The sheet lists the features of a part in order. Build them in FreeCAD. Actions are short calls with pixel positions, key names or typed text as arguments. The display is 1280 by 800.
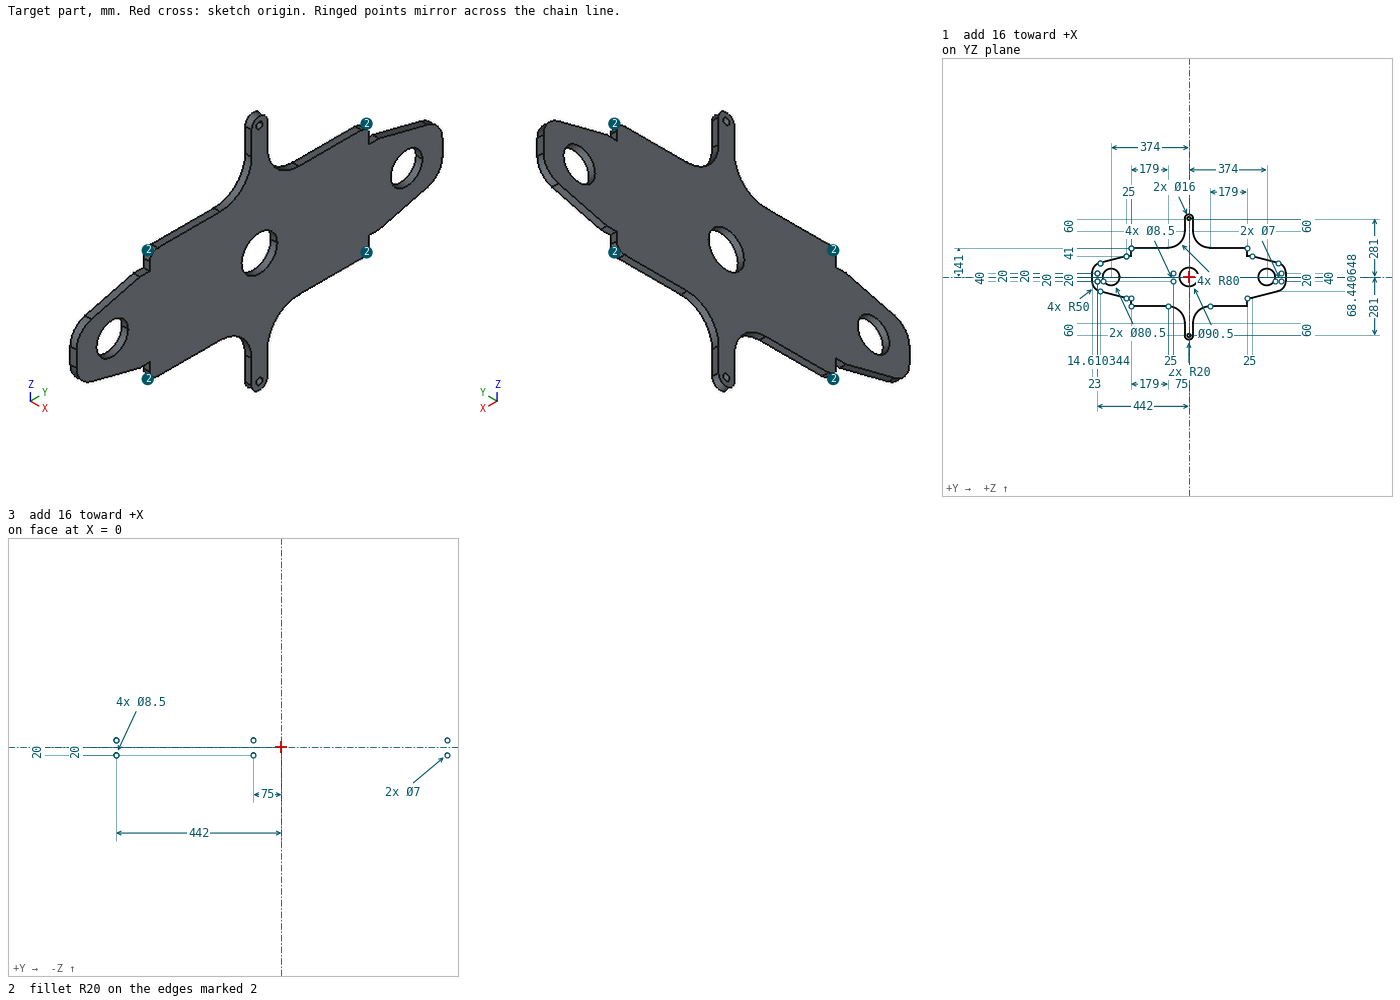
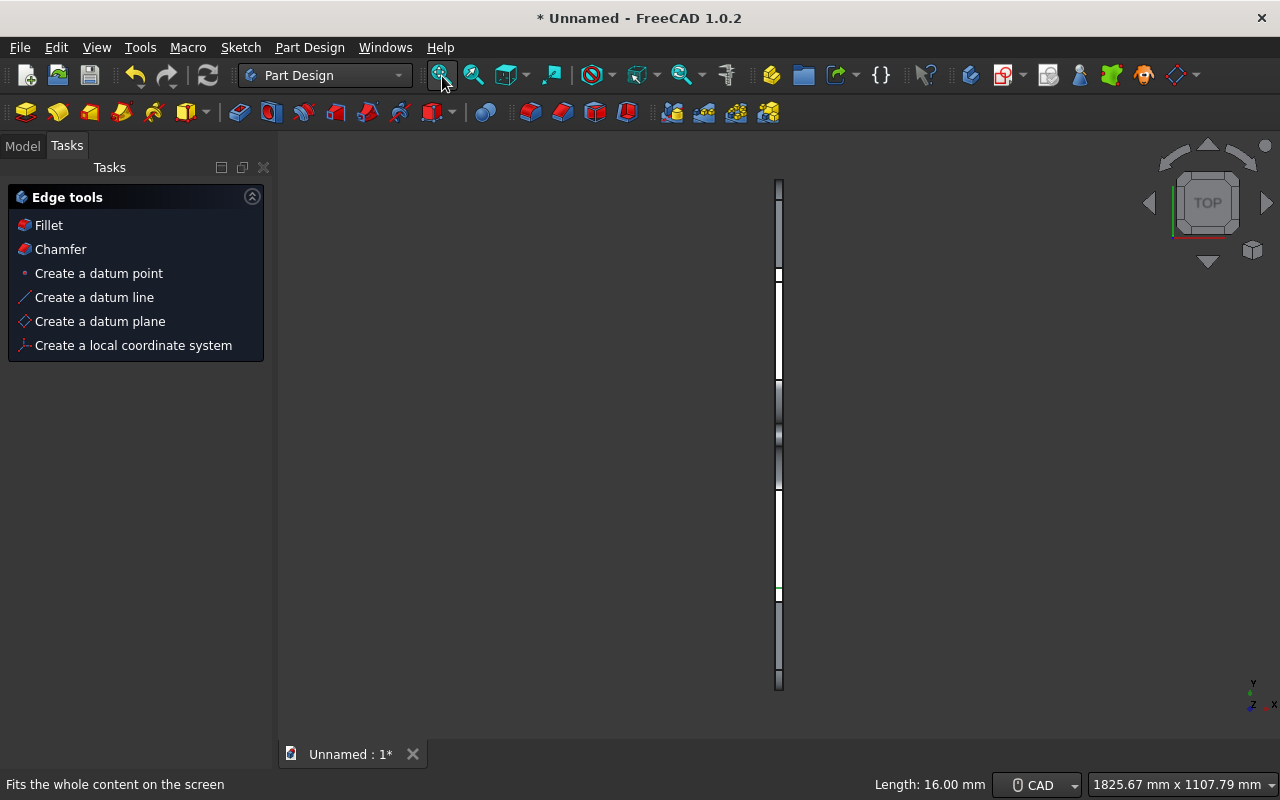
scroll(779, 281, up, 8)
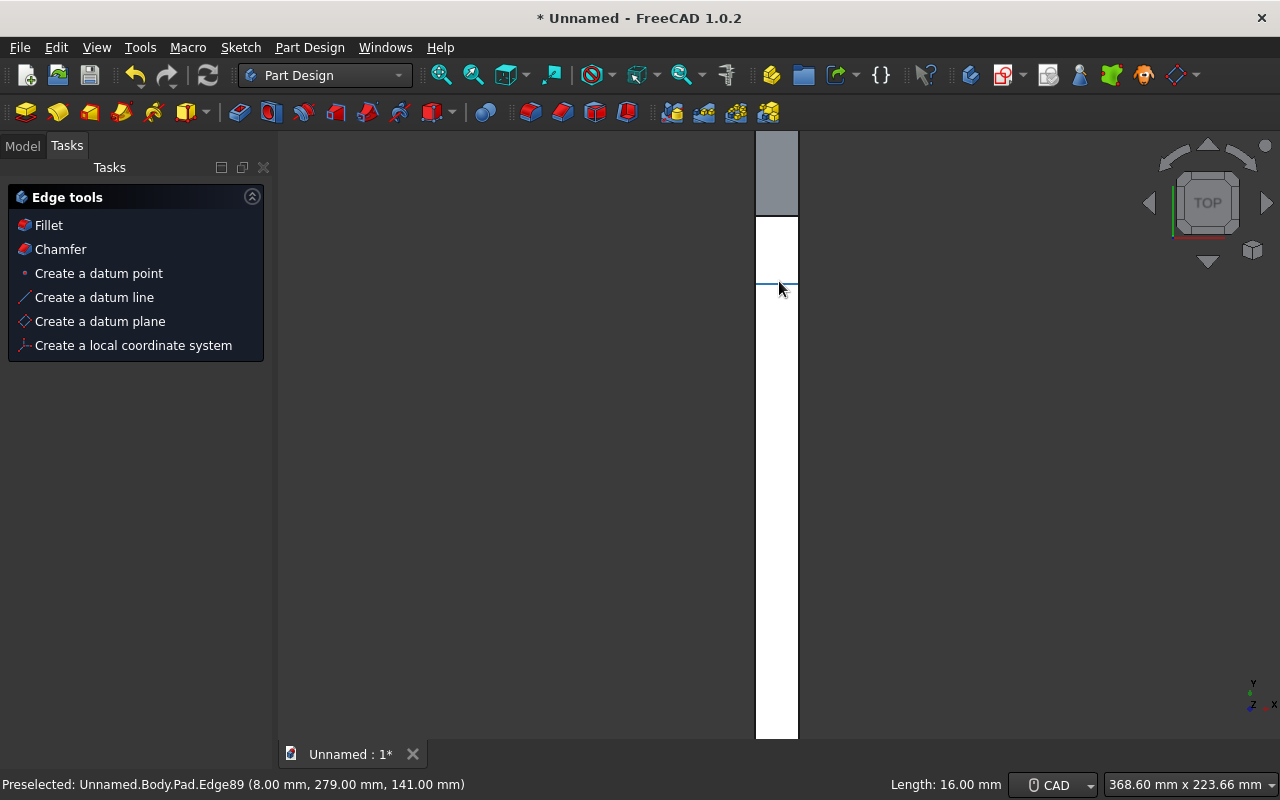
click(777, 283, ctrl)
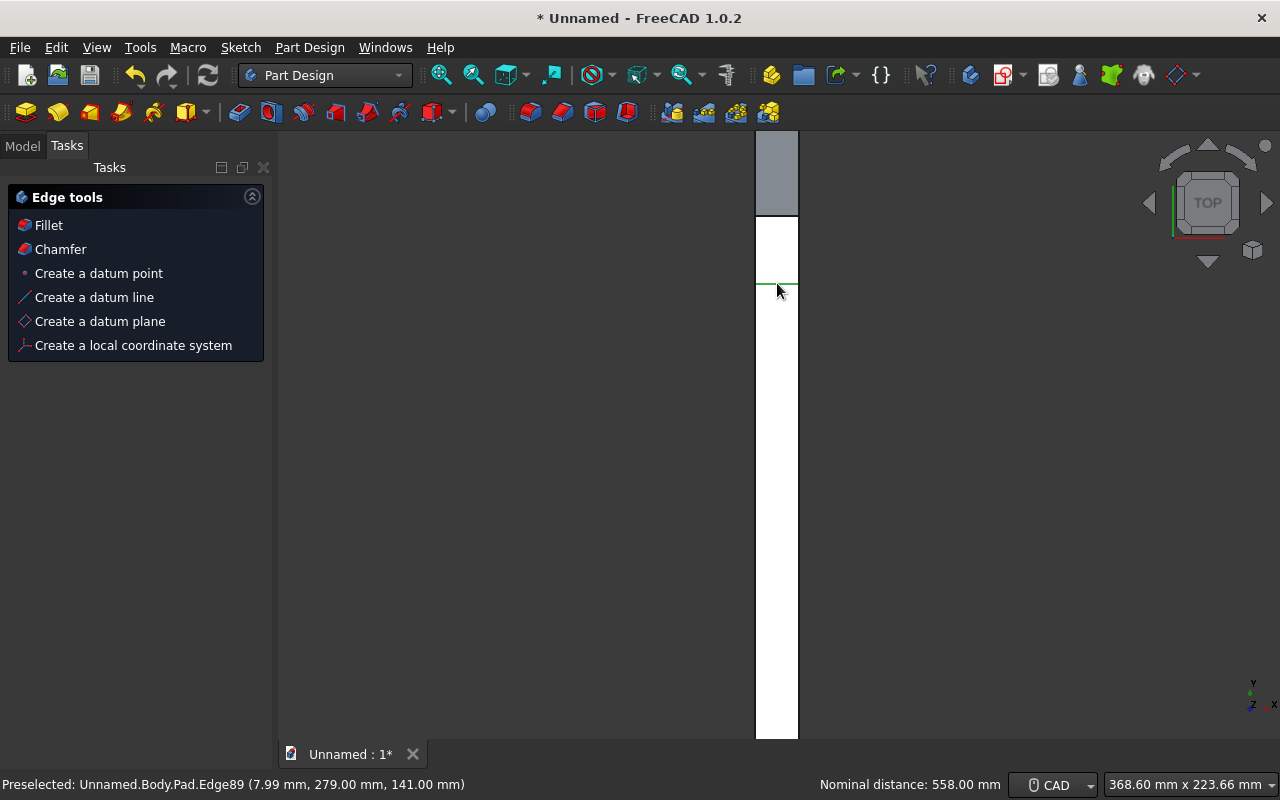
click(442, 76)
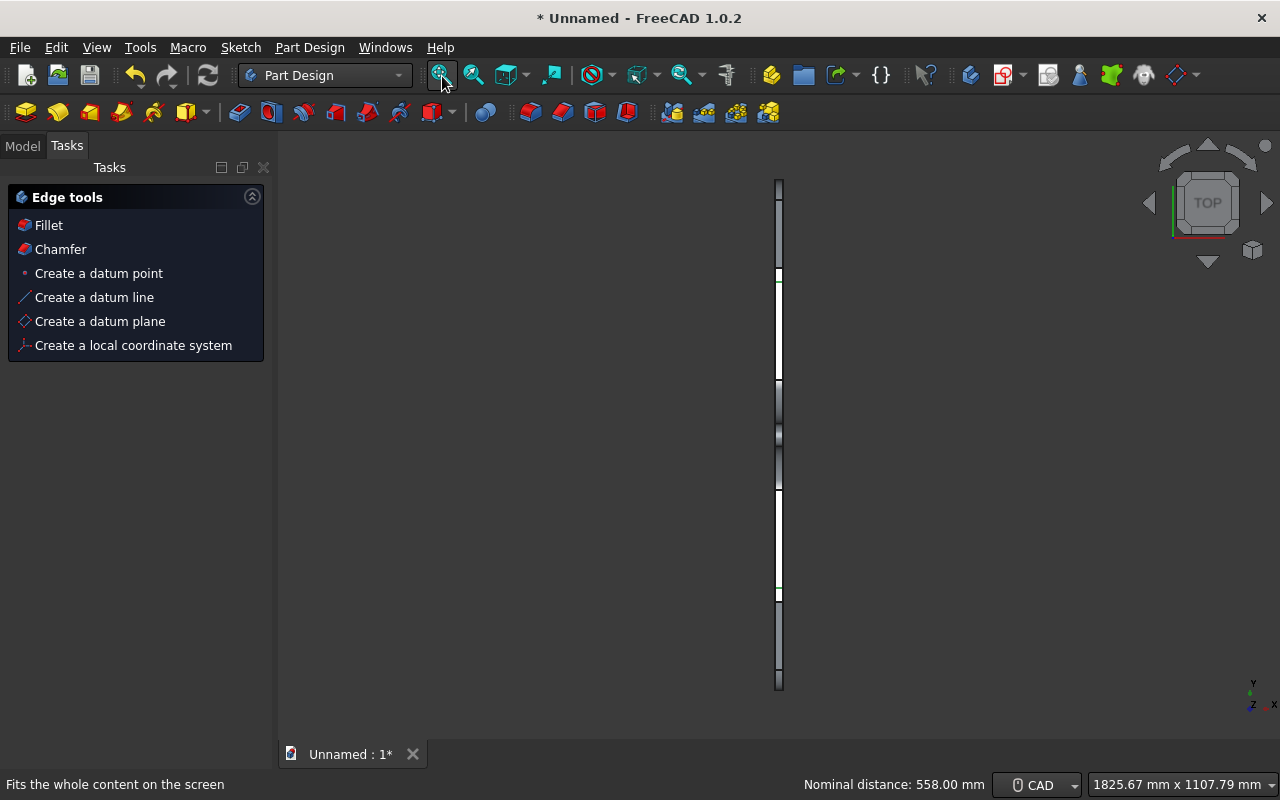
key(1)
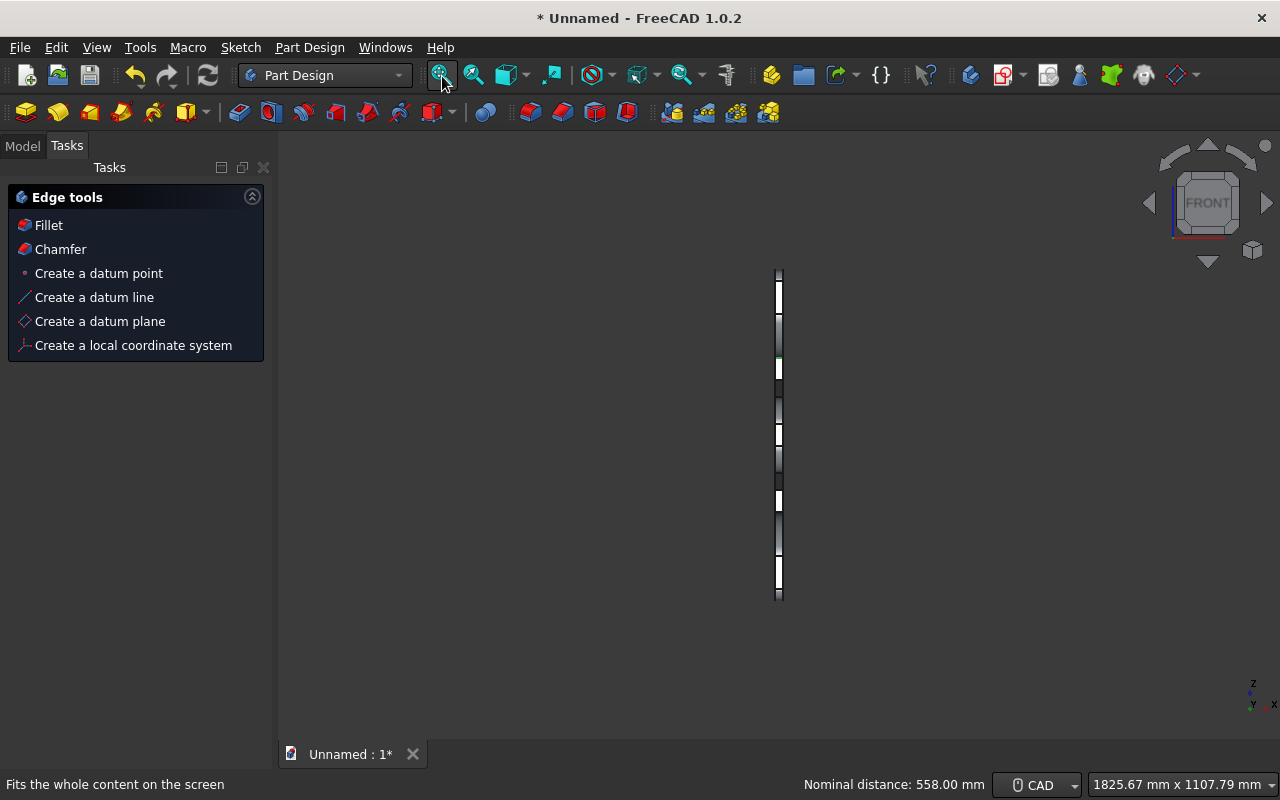
scroll(779, 511, up, 8)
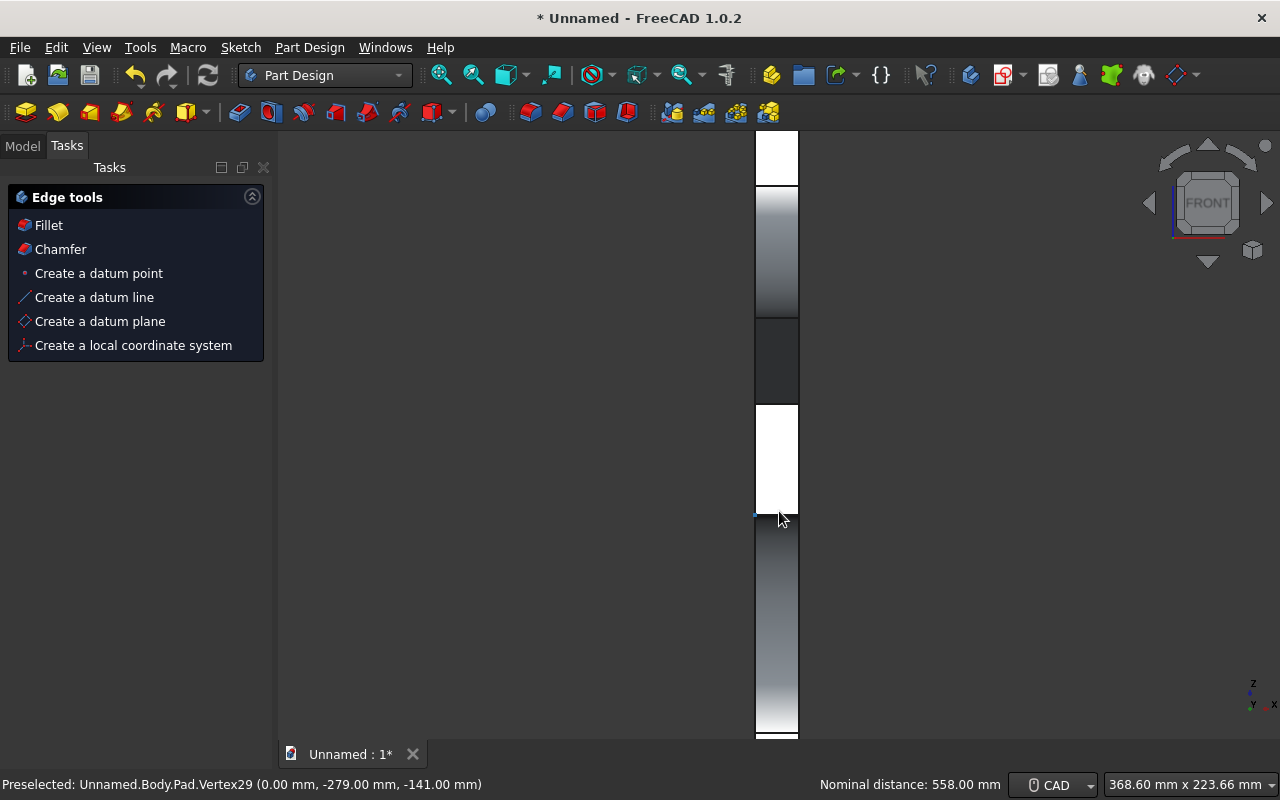
click(777, 514, ctrl)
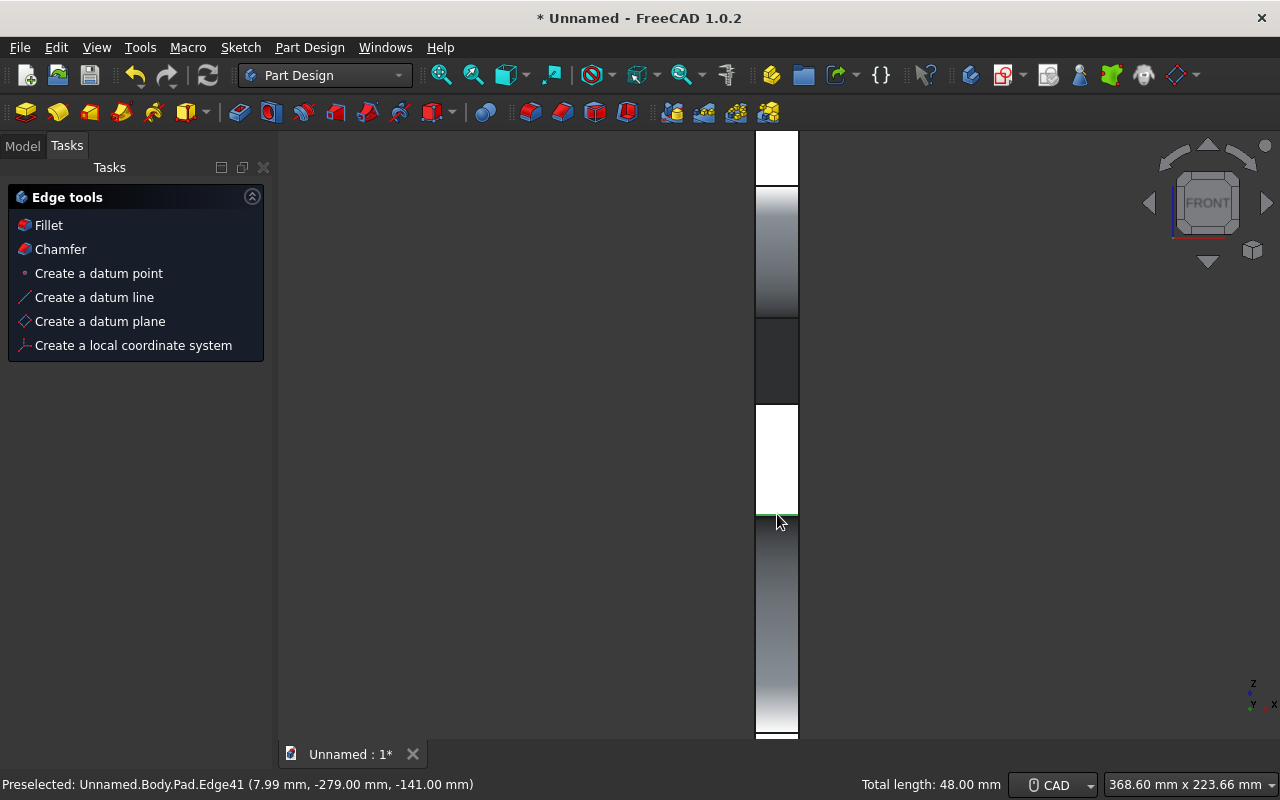
click(442, 76)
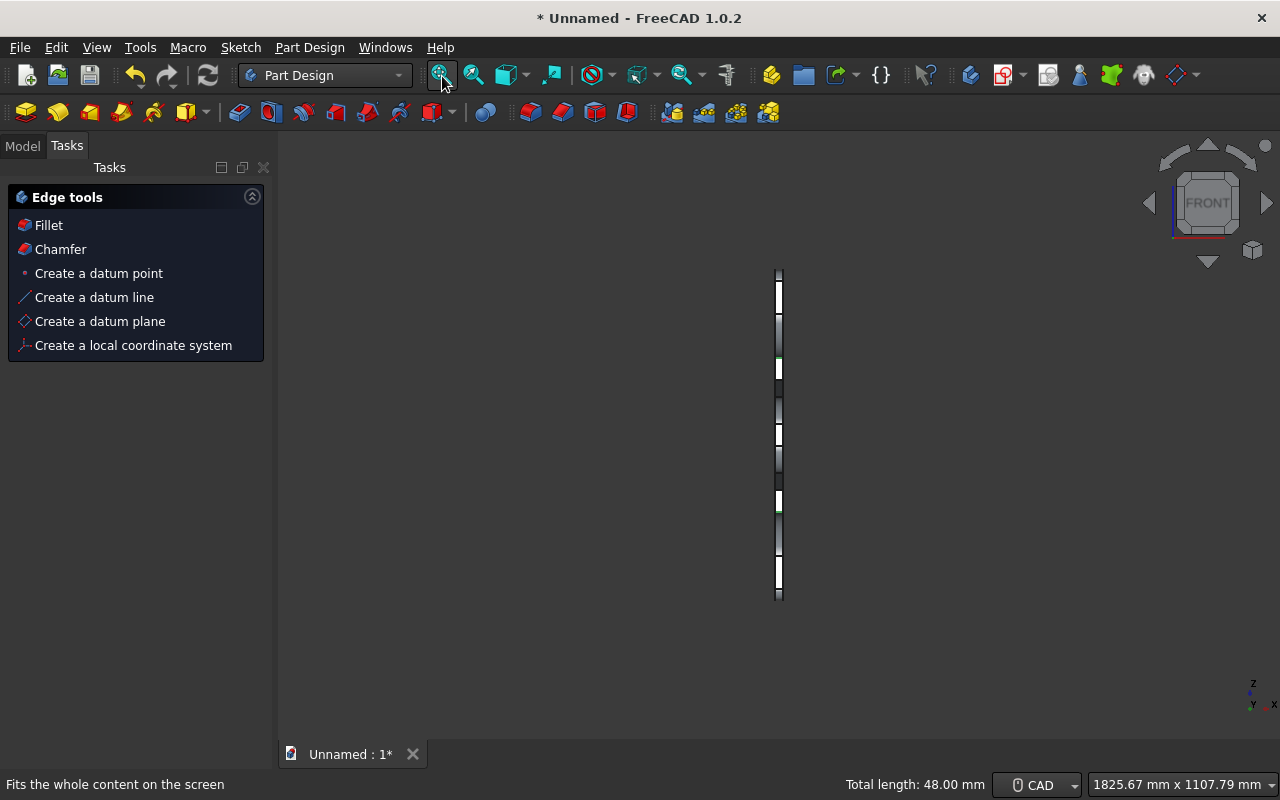
key(3)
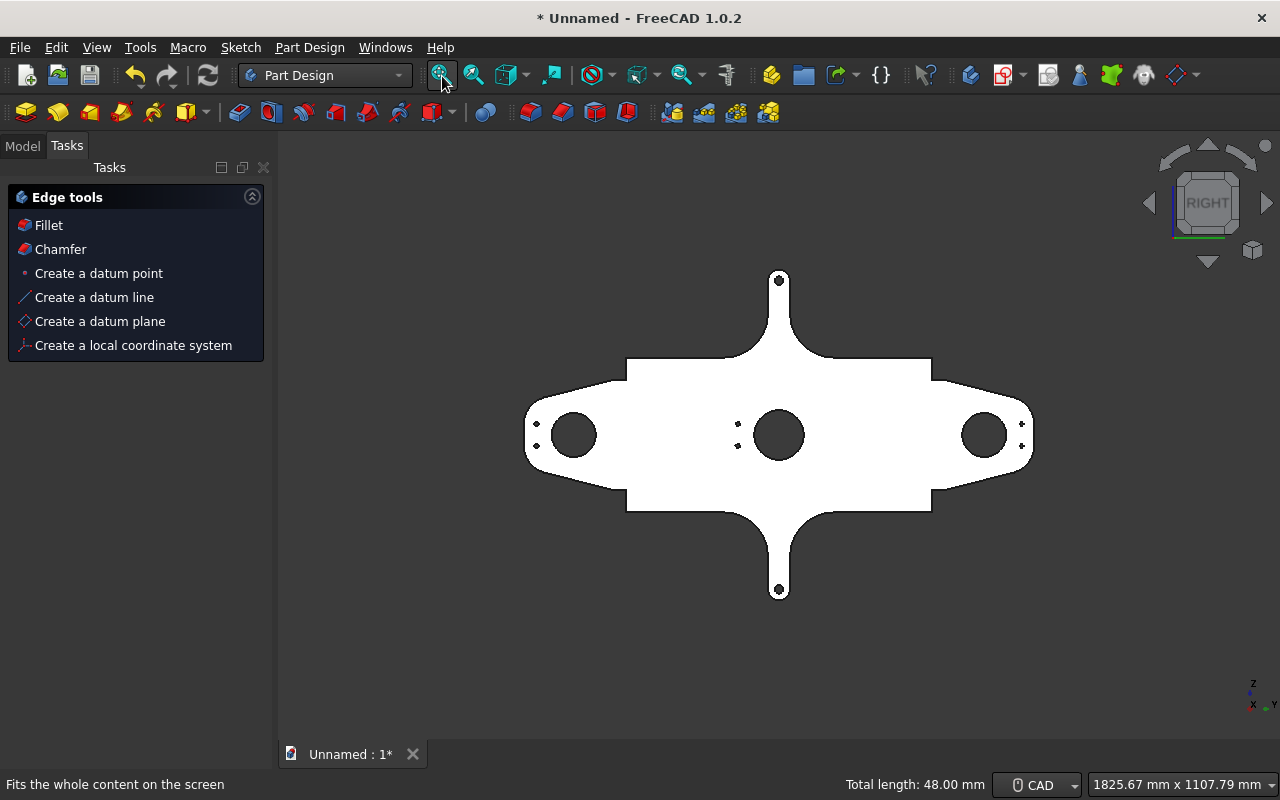
scroll(932, 511, up, 8)